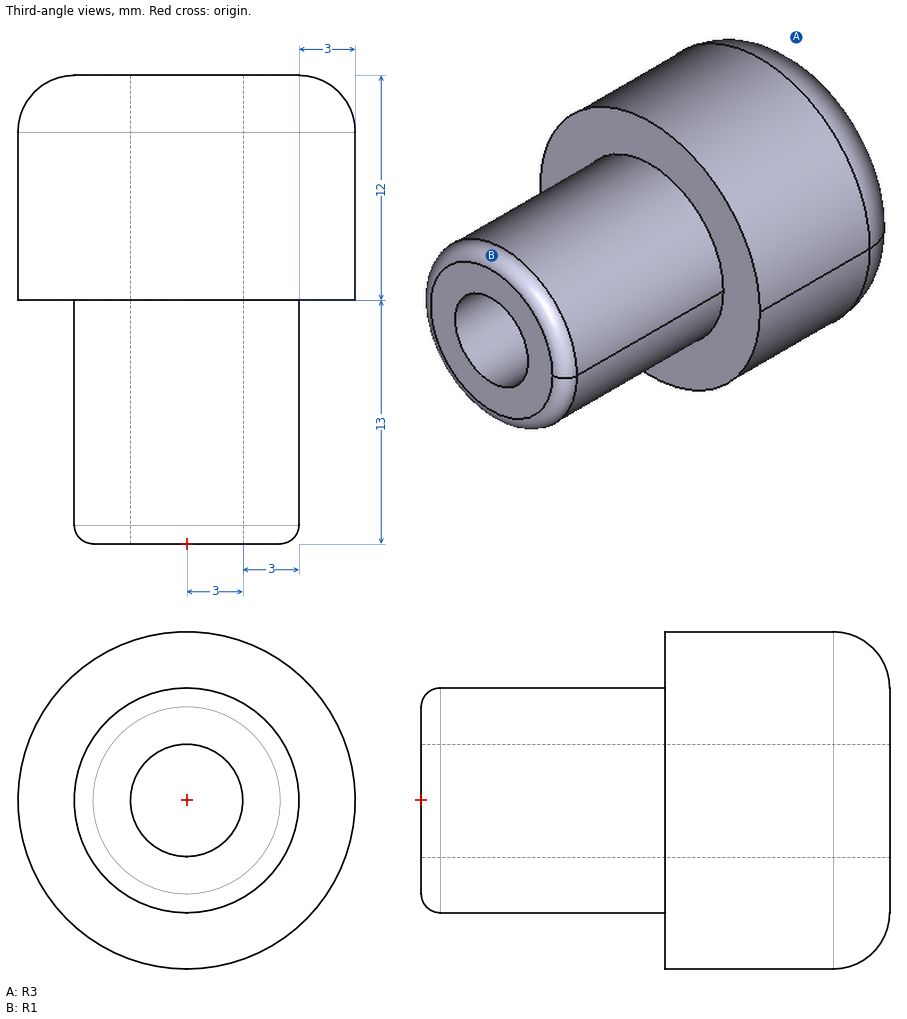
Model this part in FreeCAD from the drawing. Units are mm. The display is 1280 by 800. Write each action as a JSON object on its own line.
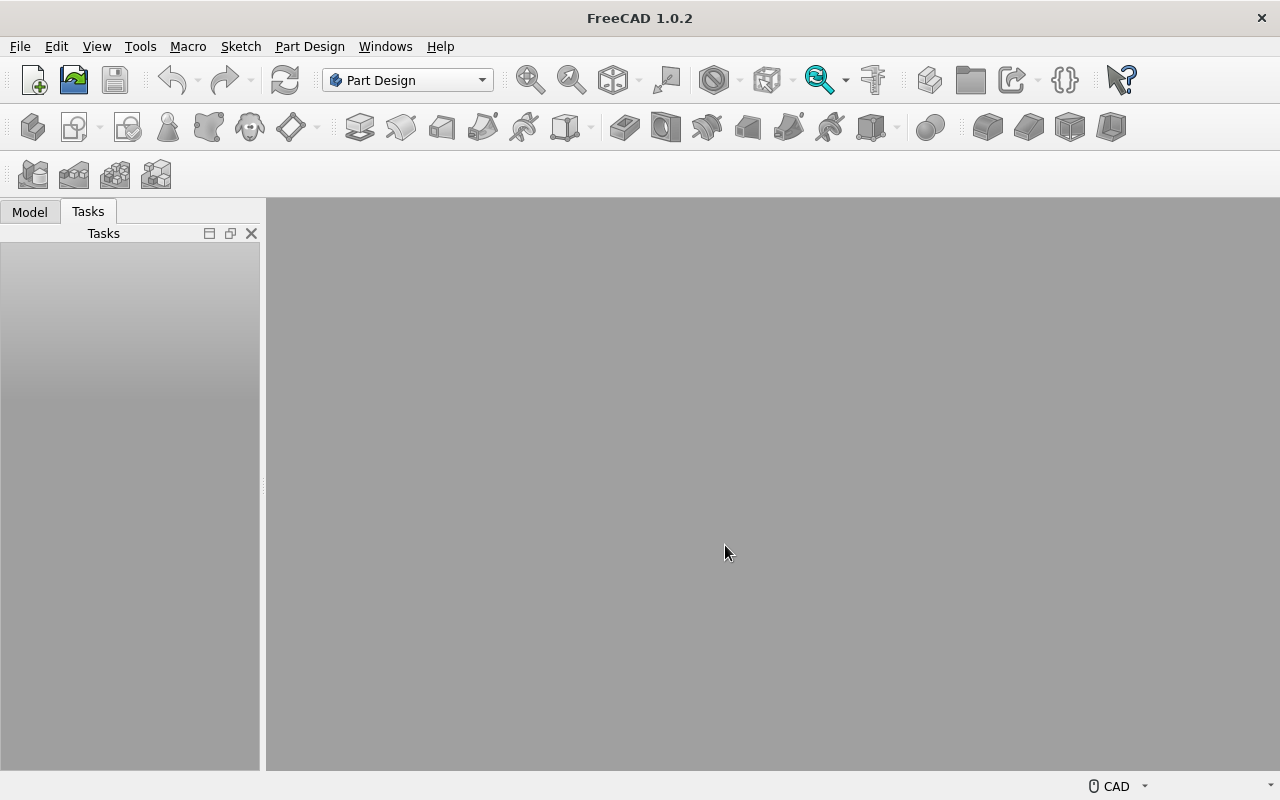
{"action": "left_click", "coordinate": [33, 80]}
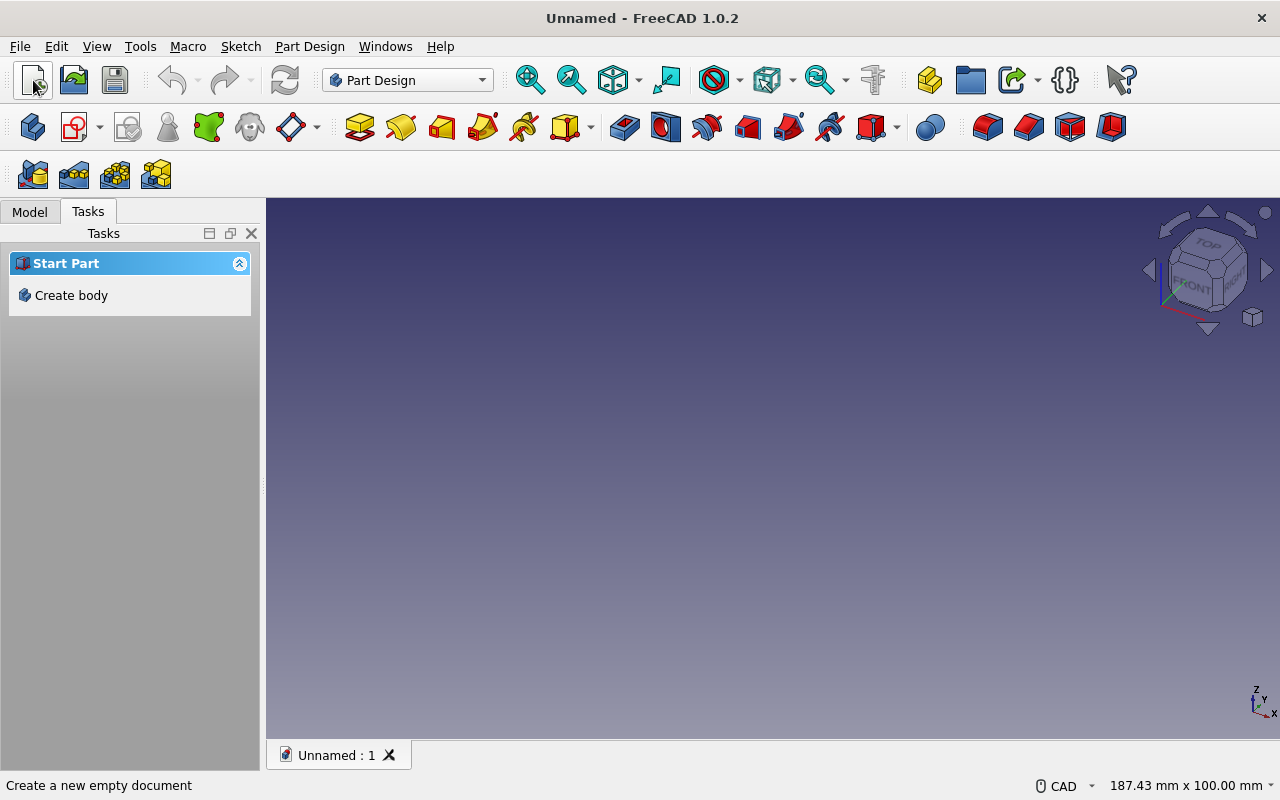
{"action": "left_click", "coordinate": [74, 128]}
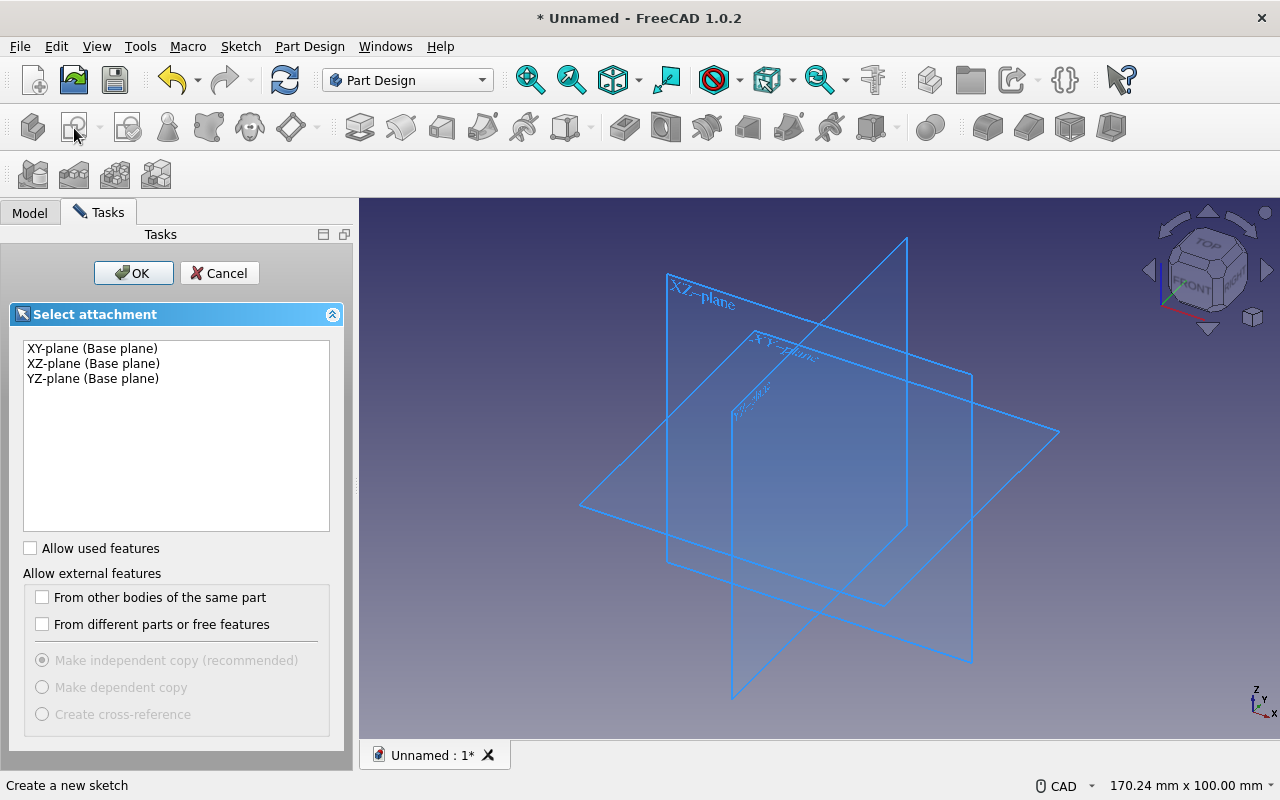
{"action": "left_click", "coordinate": [84, 348]}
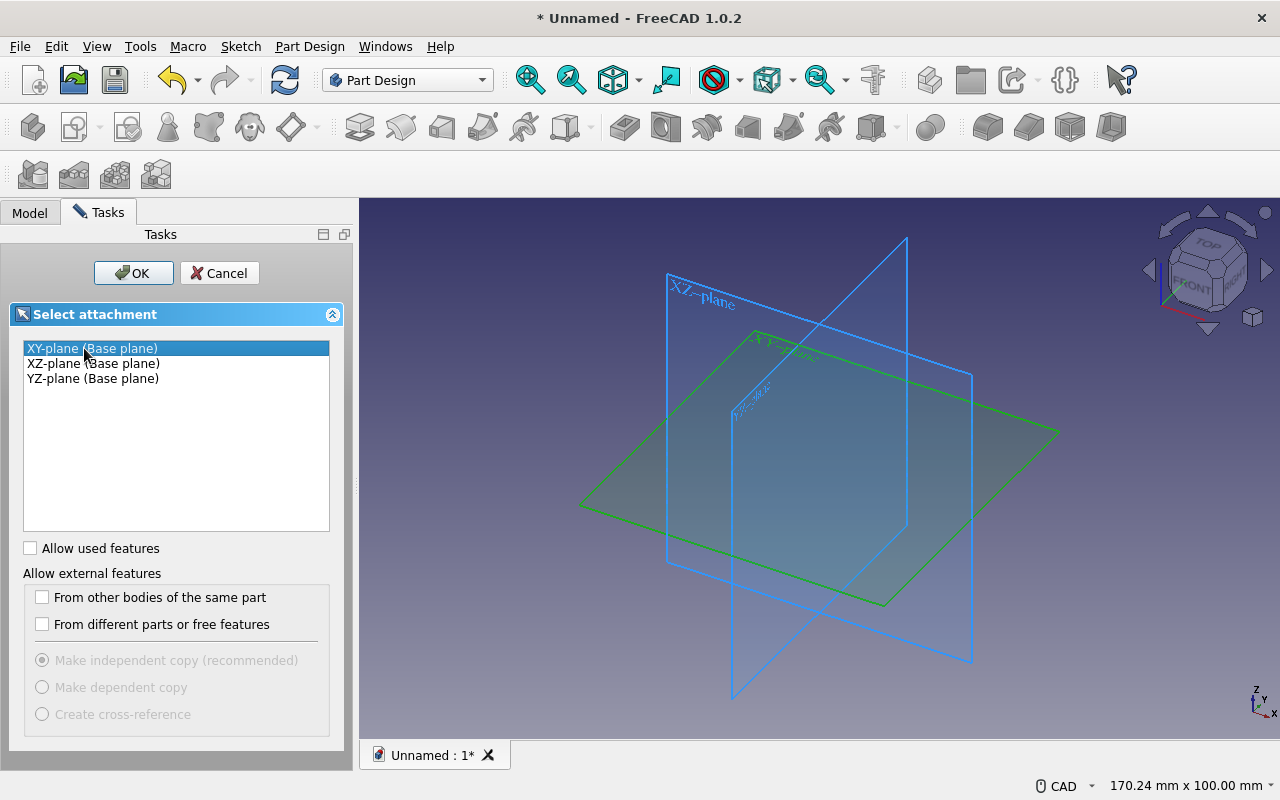
{"action": "left_click", "coordinate": [134, 273]}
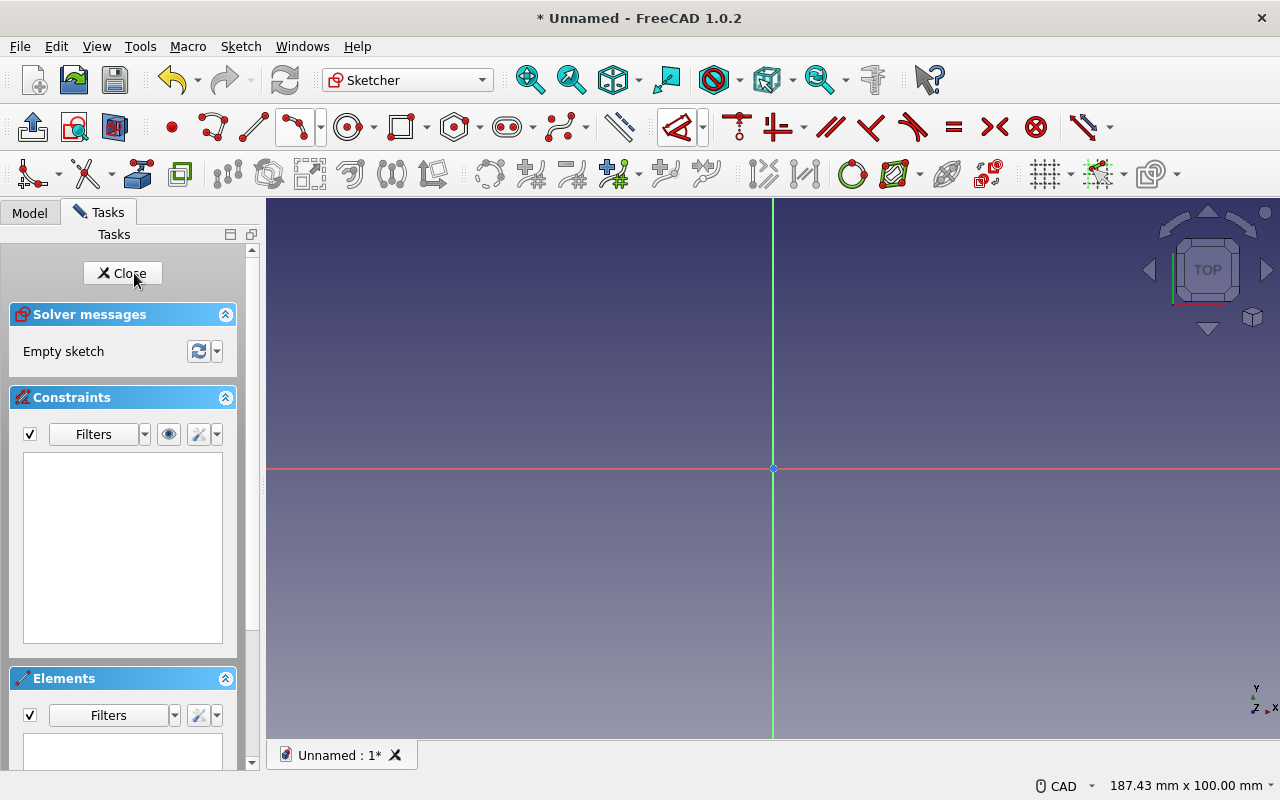
{"action": "scroll", "coordinate": [851, 362], "scroll_direction": "up", "scroll_amount": 5}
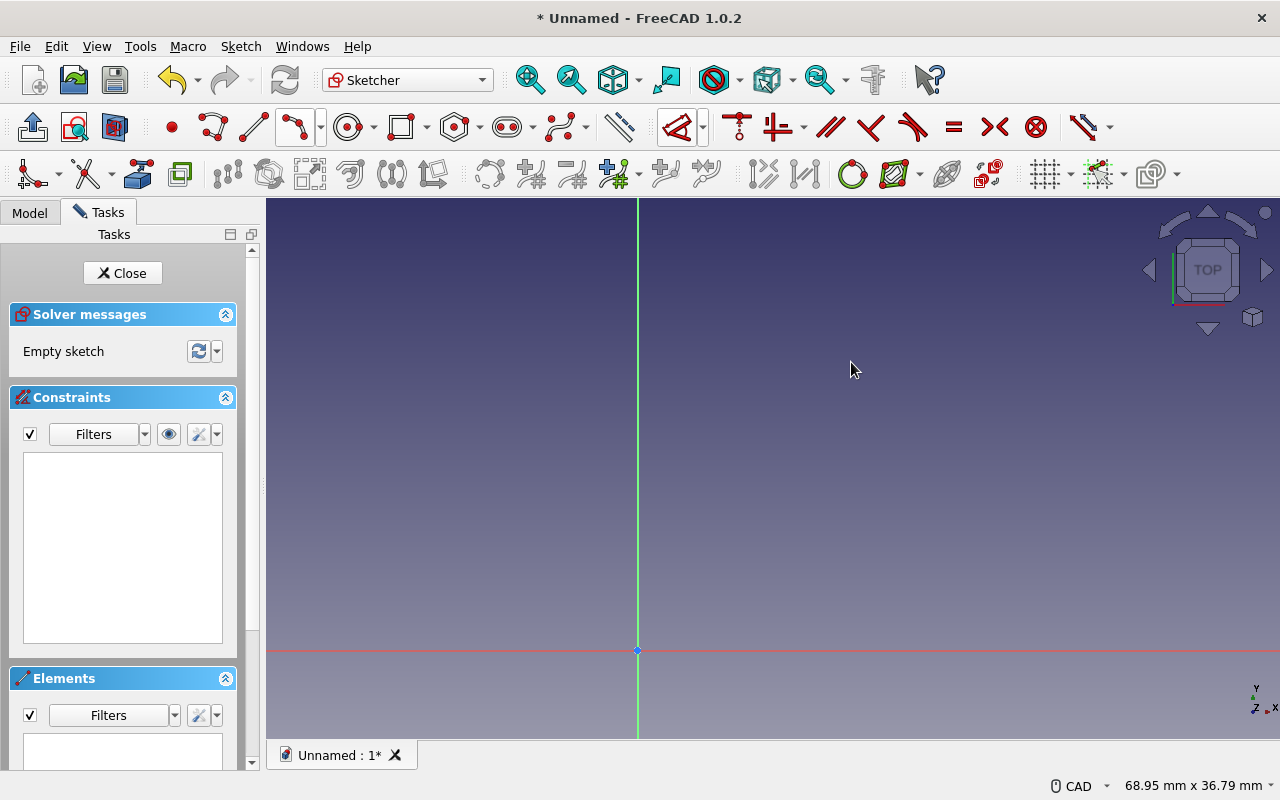
{"action": "key", "text": "g m"}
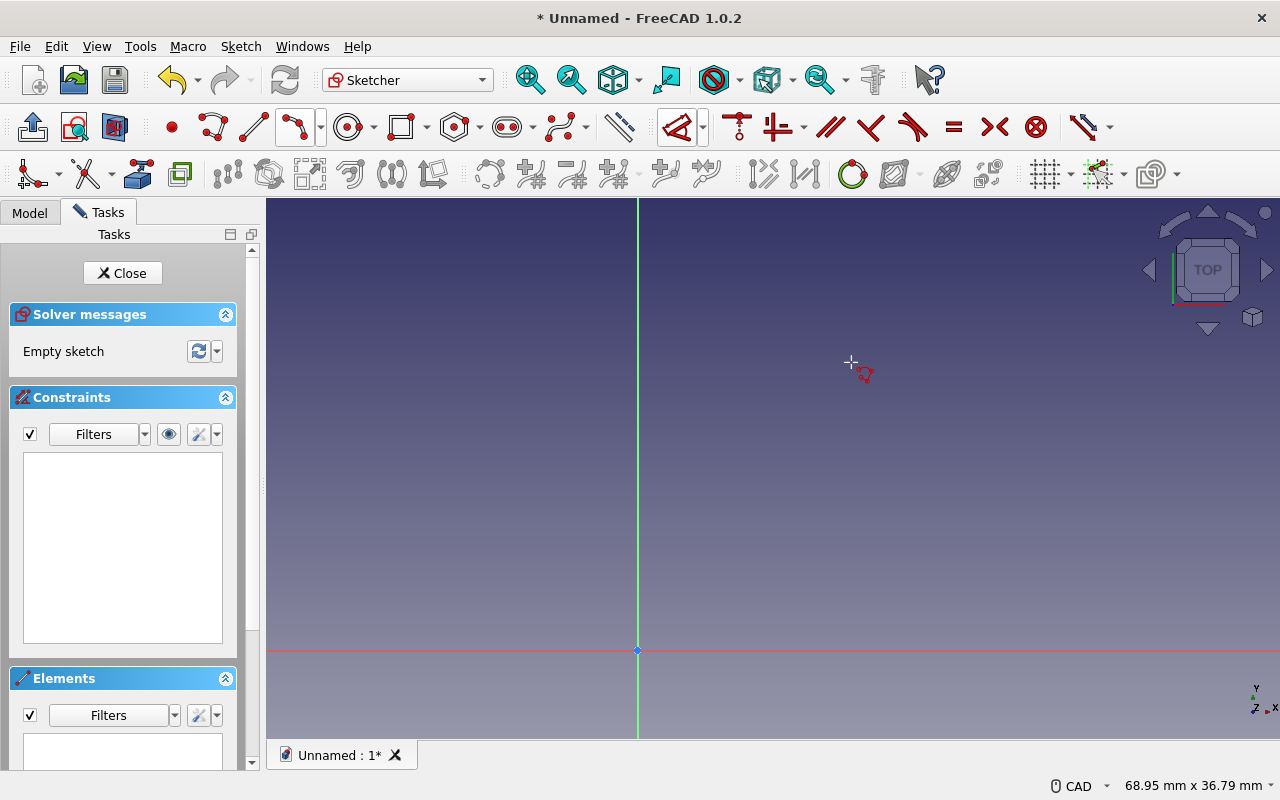
{"action": "left_click", "coordinate": [682, 651]}
{"action": "left_click", "coordinate": [726, 642]}
{"action": "left_click", "coordinate": [726, 460]}
{"action": "left_click", "coordinate": [770, 460]}
{"action": "left_click", "coordinate": [770, 283]}
{"action": "left_click", "coordinate": [682, 283]}
{"action": "left_click", "coordinate": [682, 651]}
{"action": "key", "text": "Escape"}
{"action": "key", "text": "Escape"}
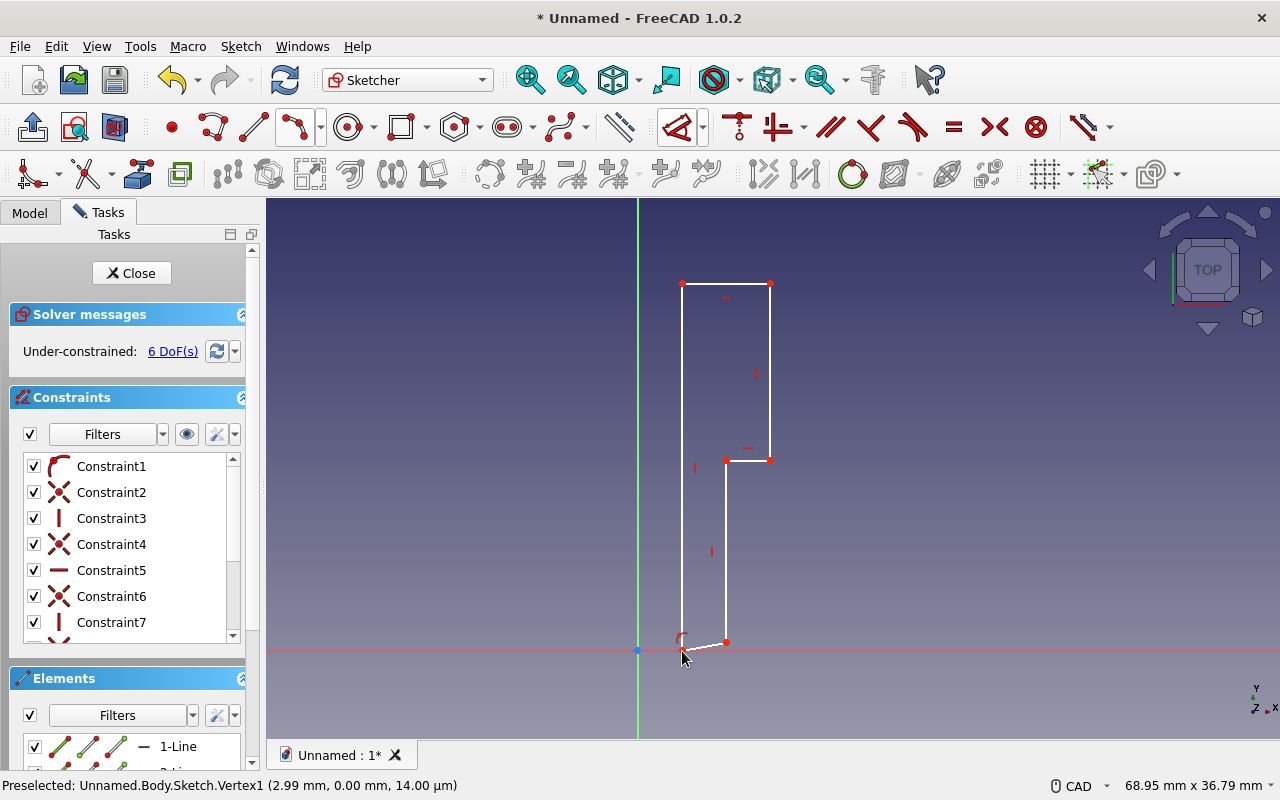
{"action": "left_click", "coordinate": [695, 649]}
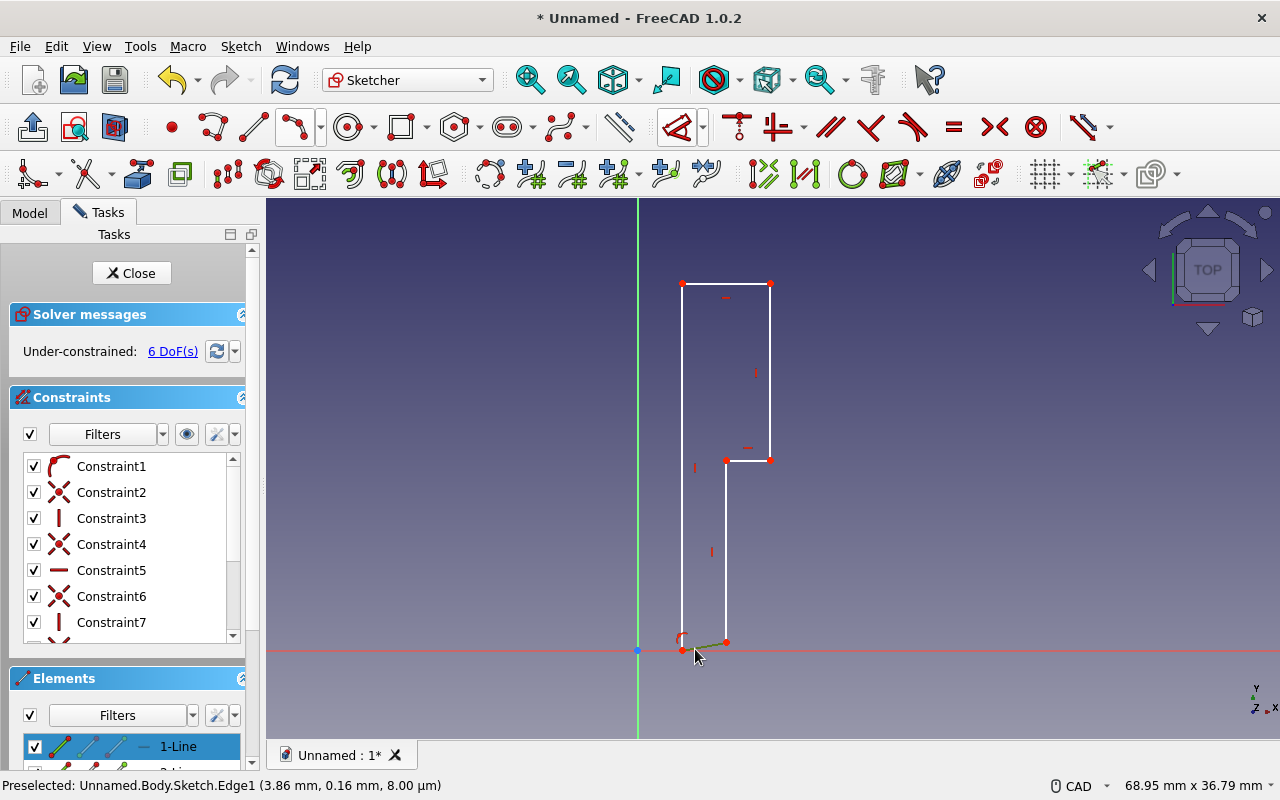
{"action": "key", "text": "h"}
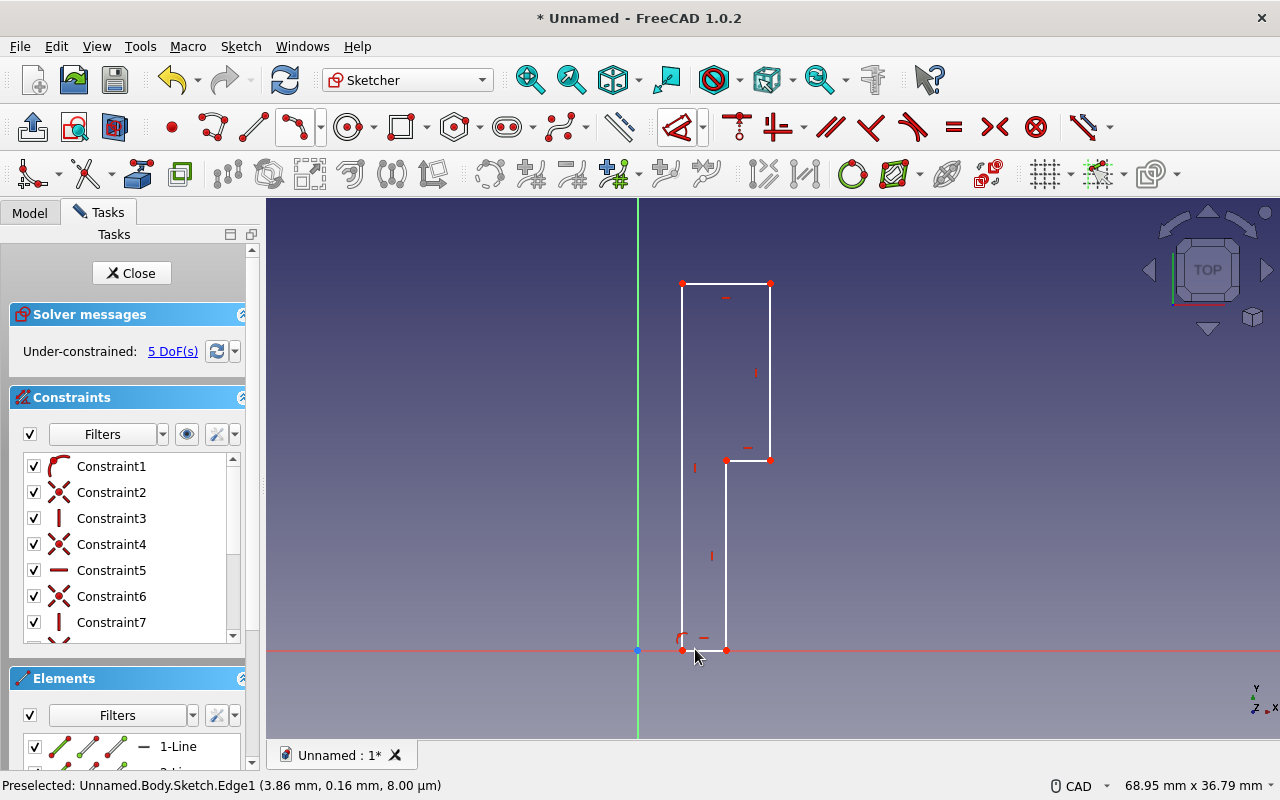
{"action": "left_click", "coordinate": [695, 651]}